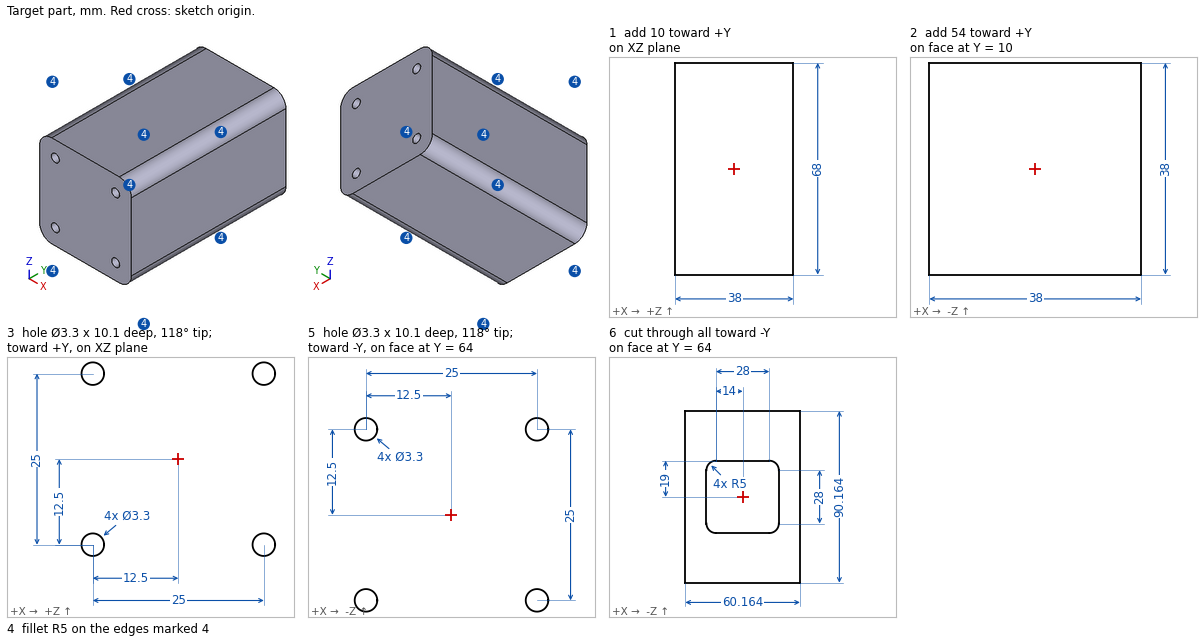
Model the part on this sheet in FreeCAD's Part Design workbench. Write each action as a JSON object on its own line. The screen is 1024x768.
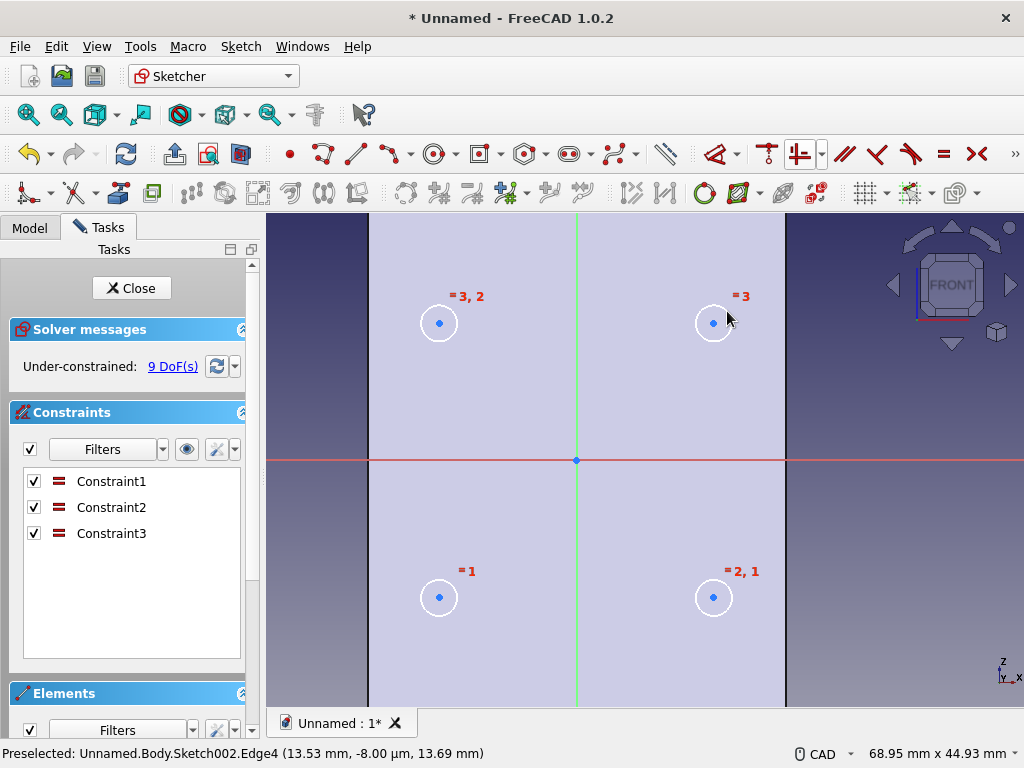
{"action": "left_click", "coordinate": [439, 598]}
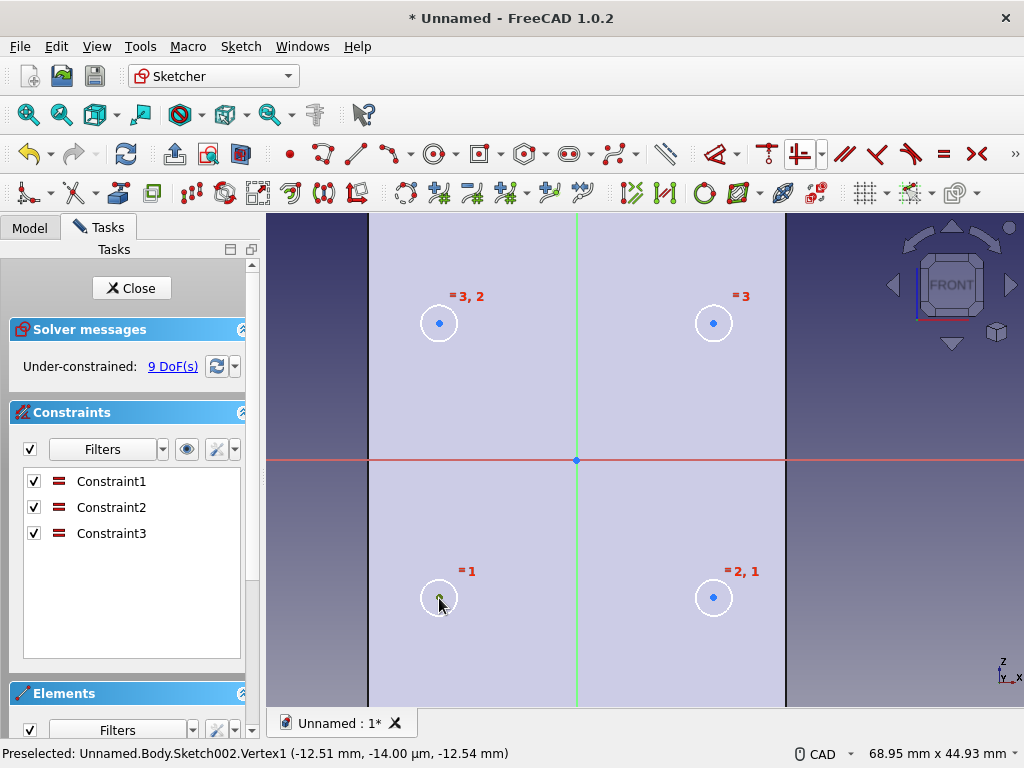
{"action": "left_click", "coordinate": [714, 598]}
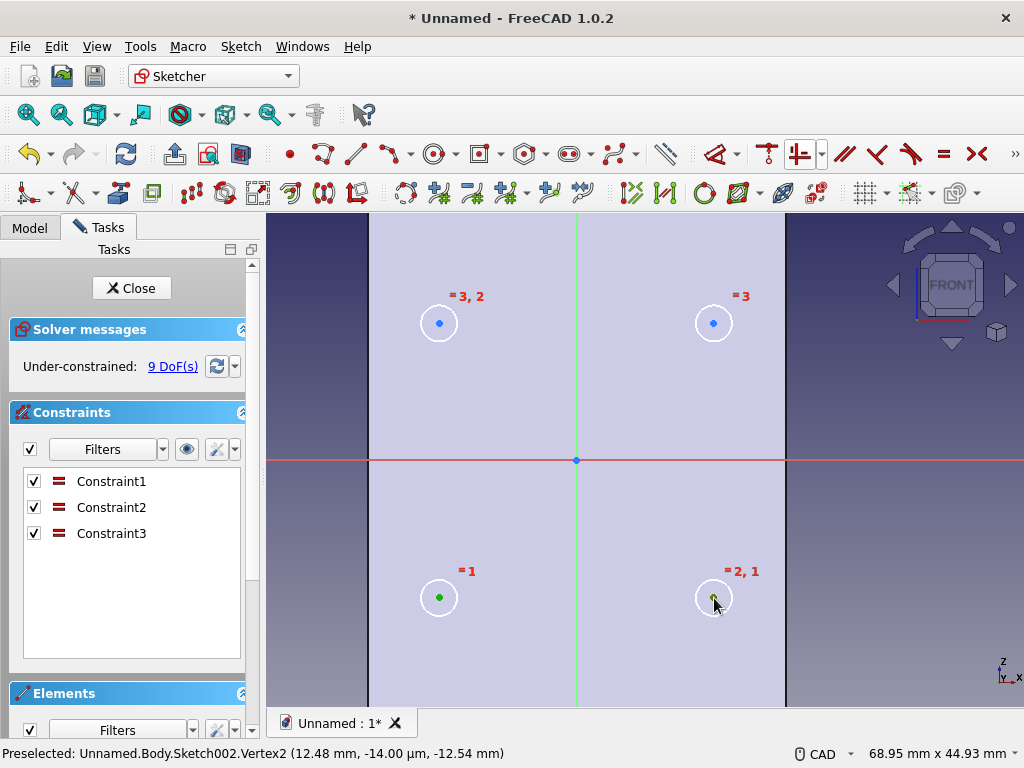
{"action": "left_click", "coordinate": [822, 154]}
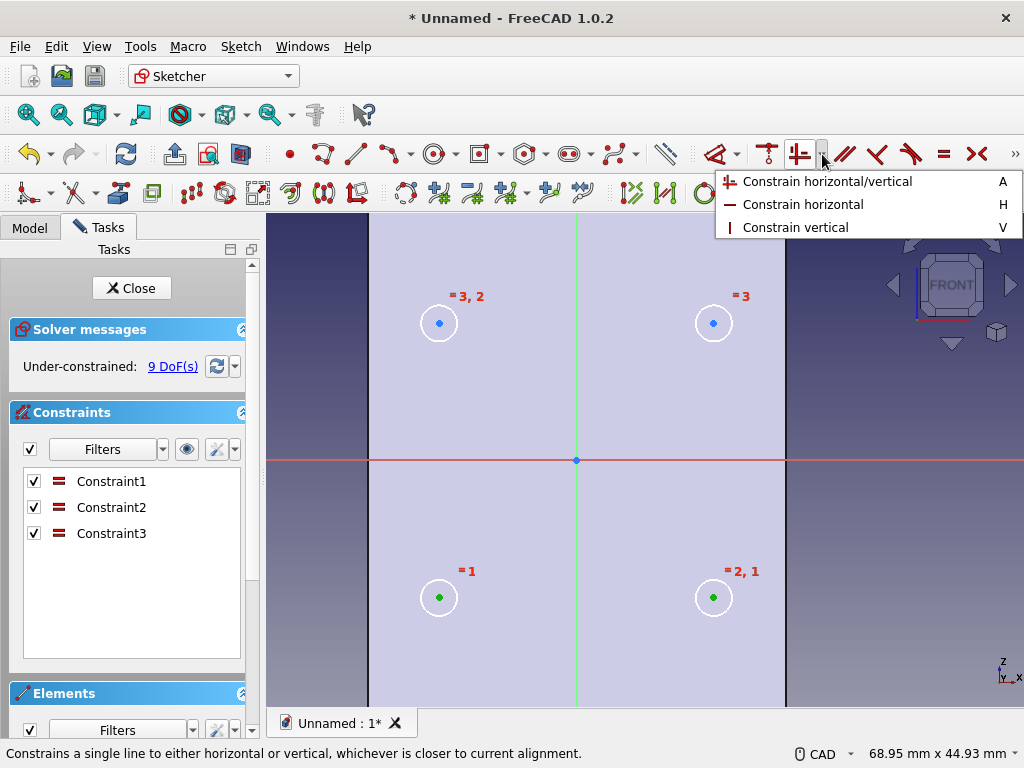
{"action": "left_click", "coordinate": [869, 204]}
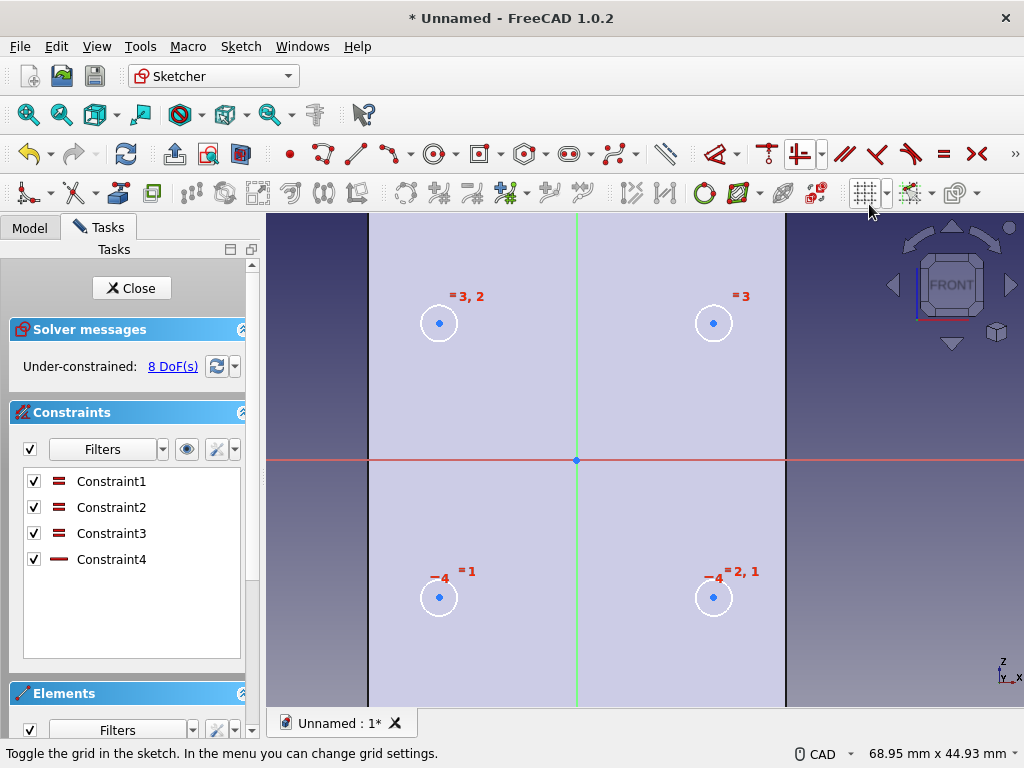
{"action": "left_click", "coordinate": [439, 598]}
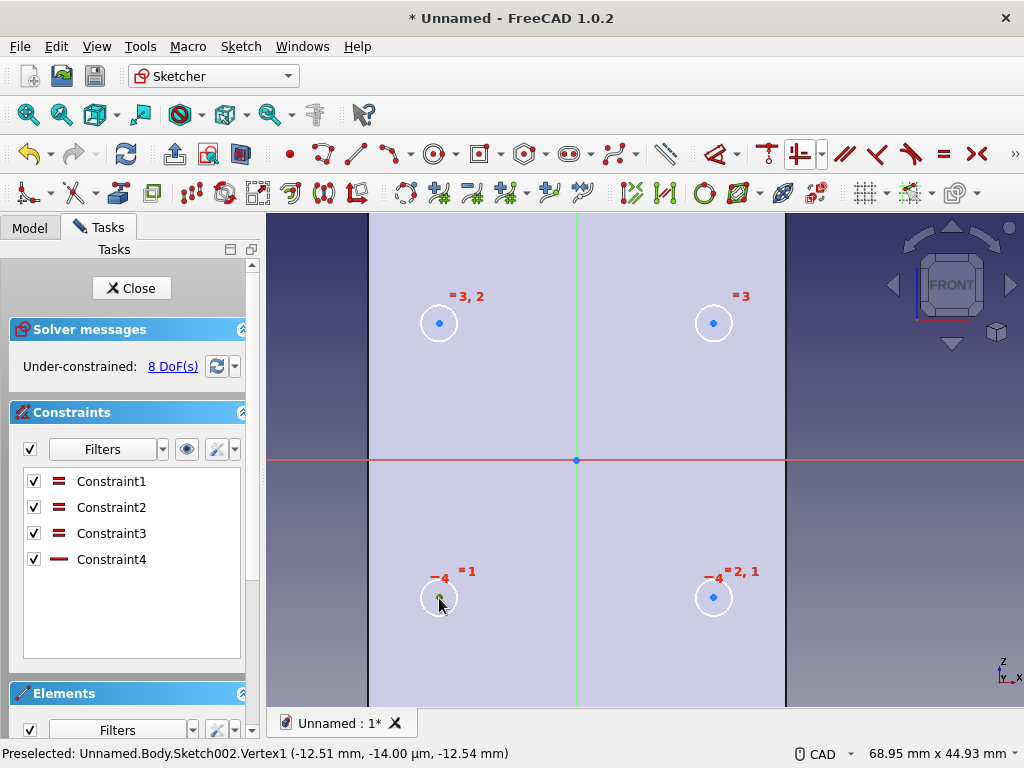
{"action": "left_click", "coordinate": [439, 323]}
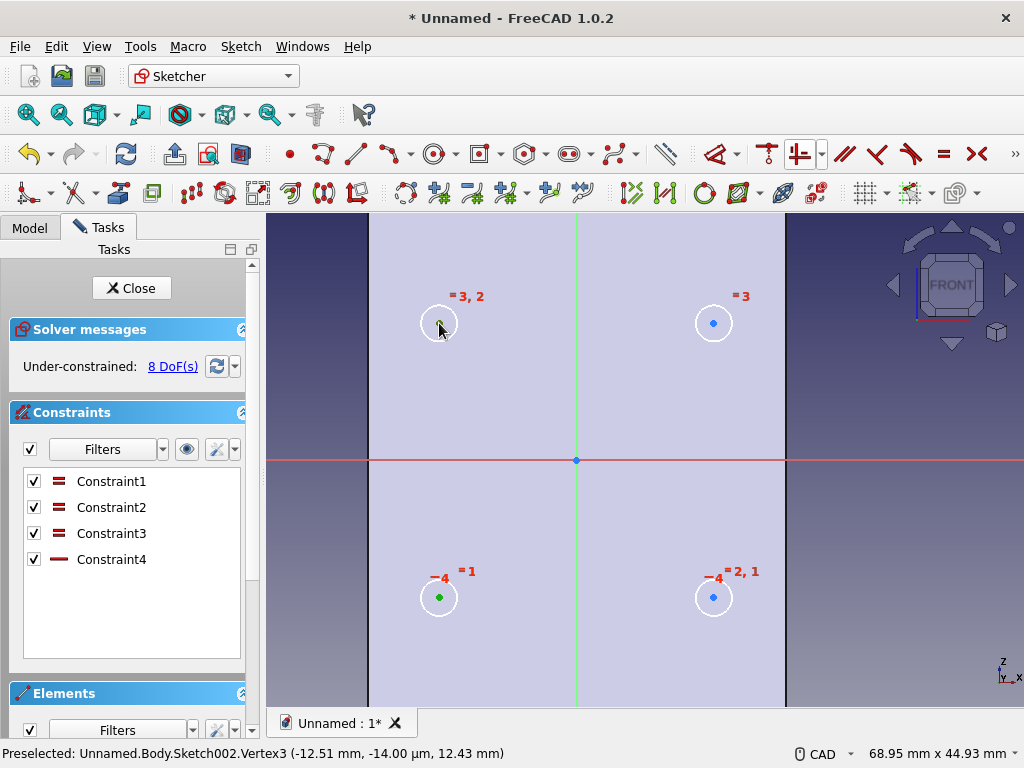
{"action": "left_click", "coordinate": [822, 154]}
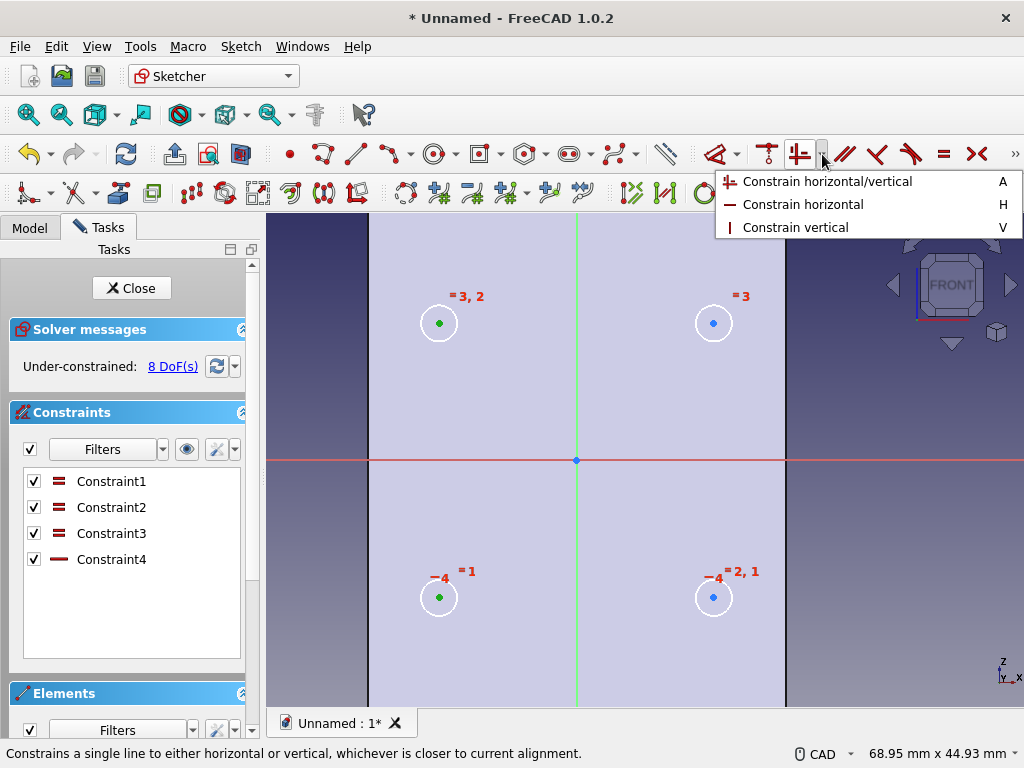
{"action": "left_click", "coordinate": [869, 228]}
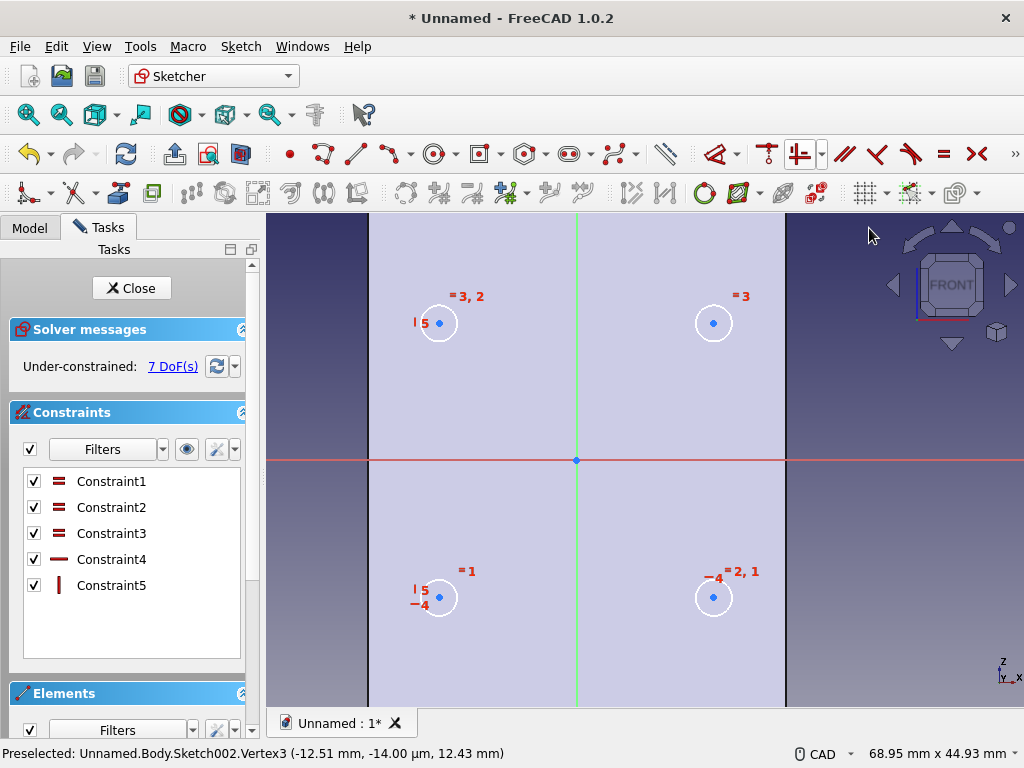
{"action": "left_click", "coordinate": [714, 598]}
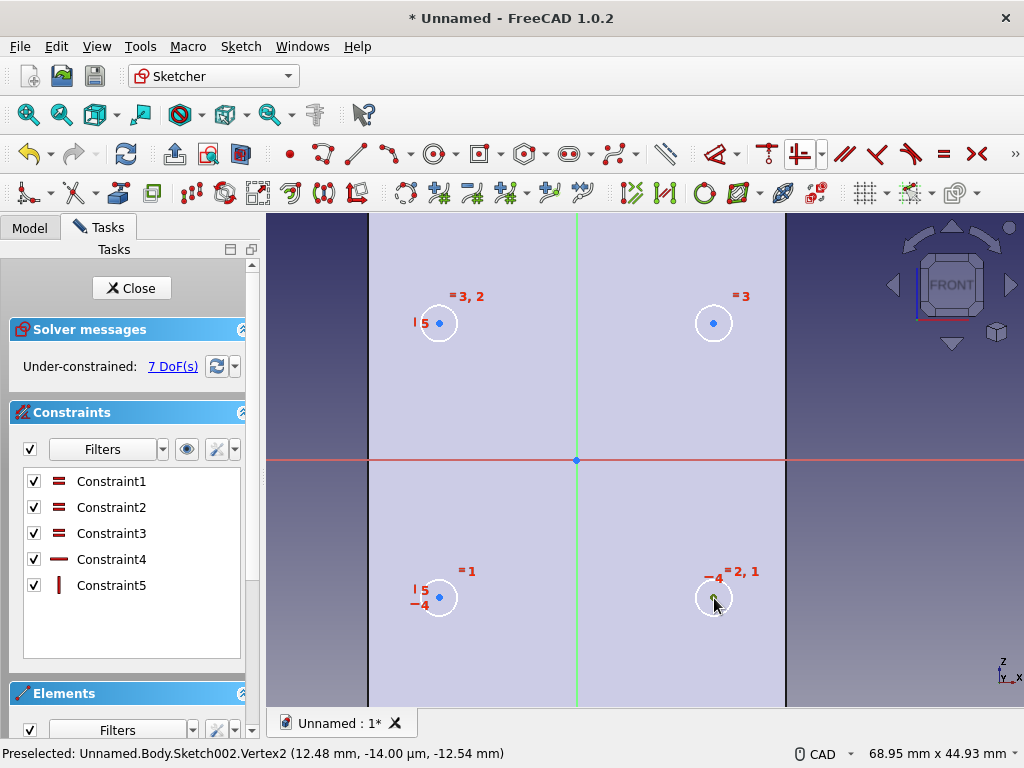
{"action": "left_click", "coordinate": [714, 323]}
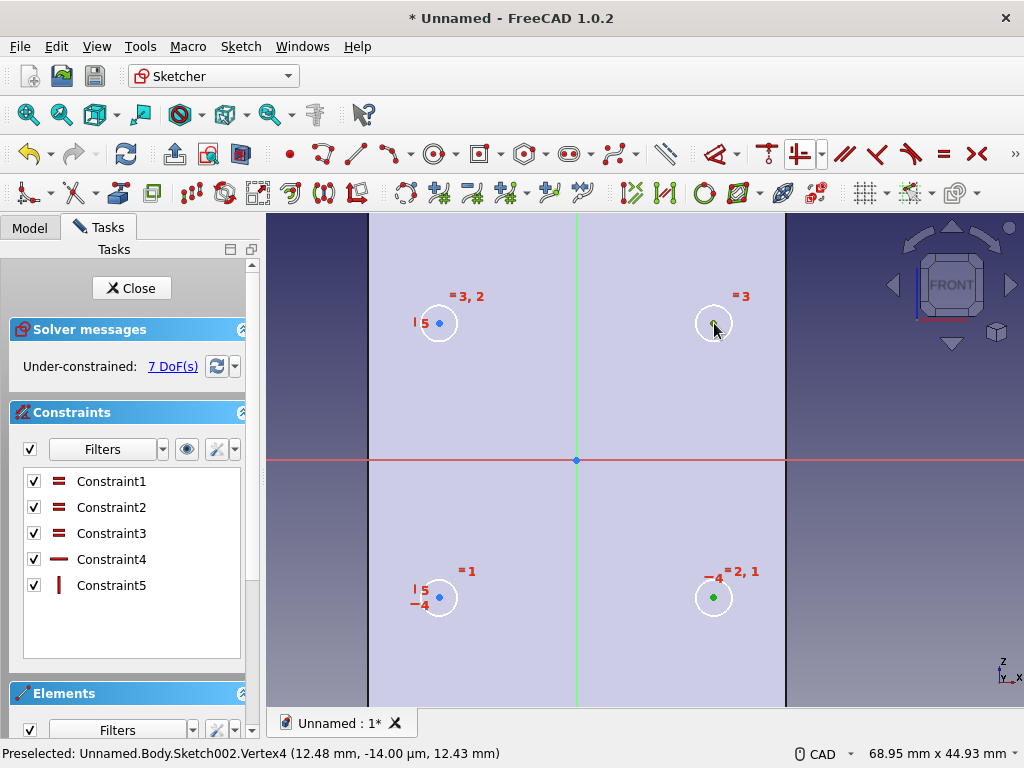
{"action": "key", "text": "v"}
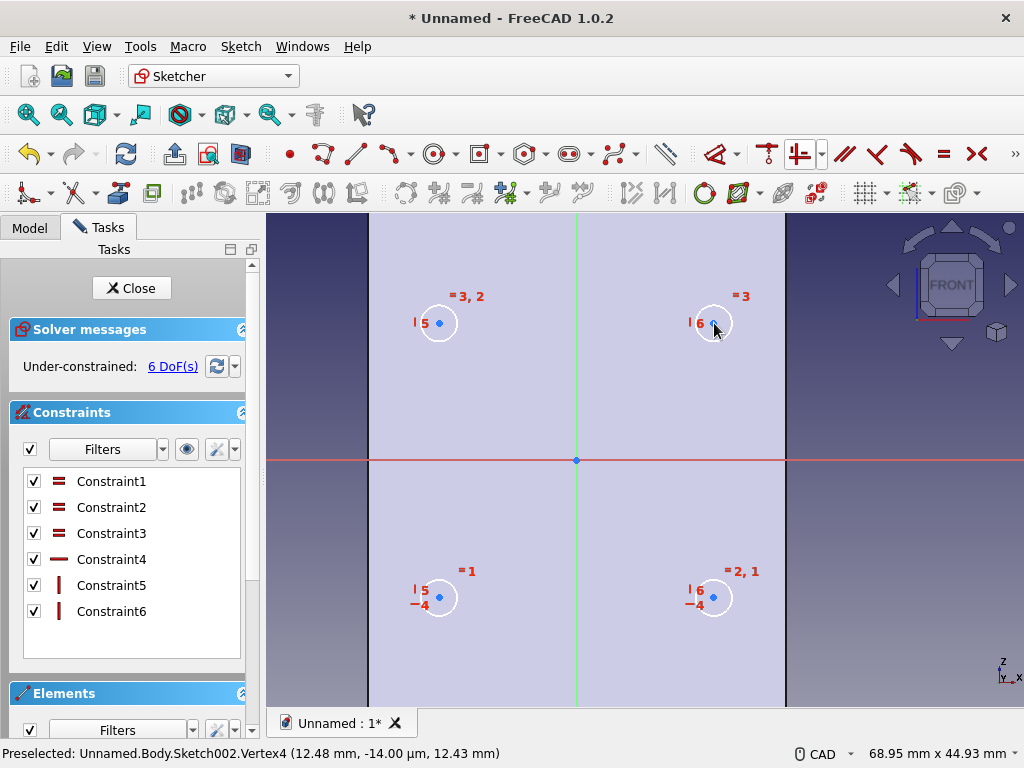
{"action": "left_click", "coordinate": [439, 323]}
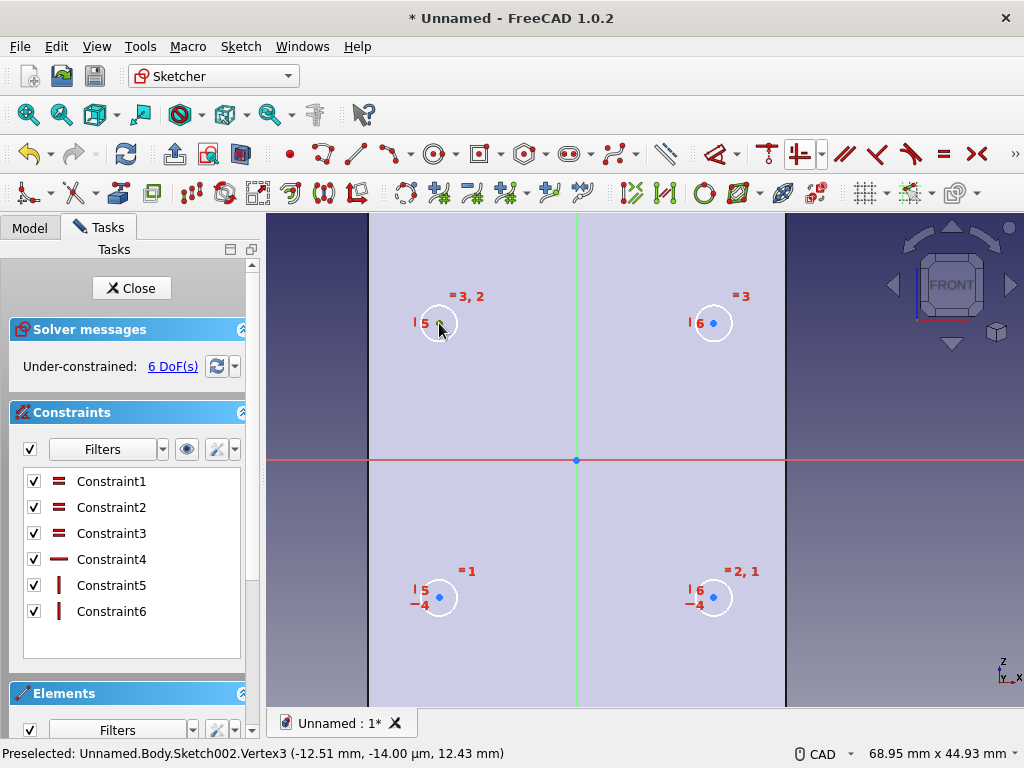
{"action": "left_click", "coordinate": [714, 323]}